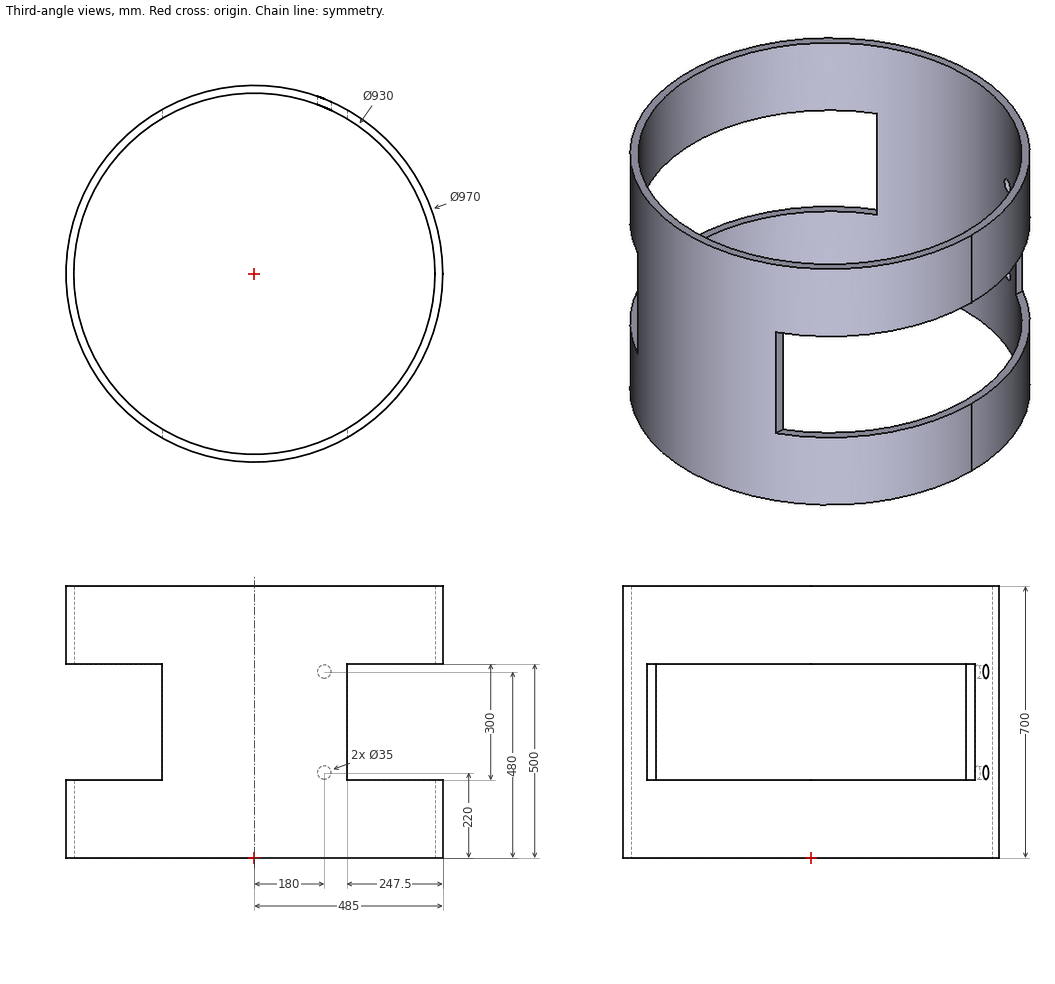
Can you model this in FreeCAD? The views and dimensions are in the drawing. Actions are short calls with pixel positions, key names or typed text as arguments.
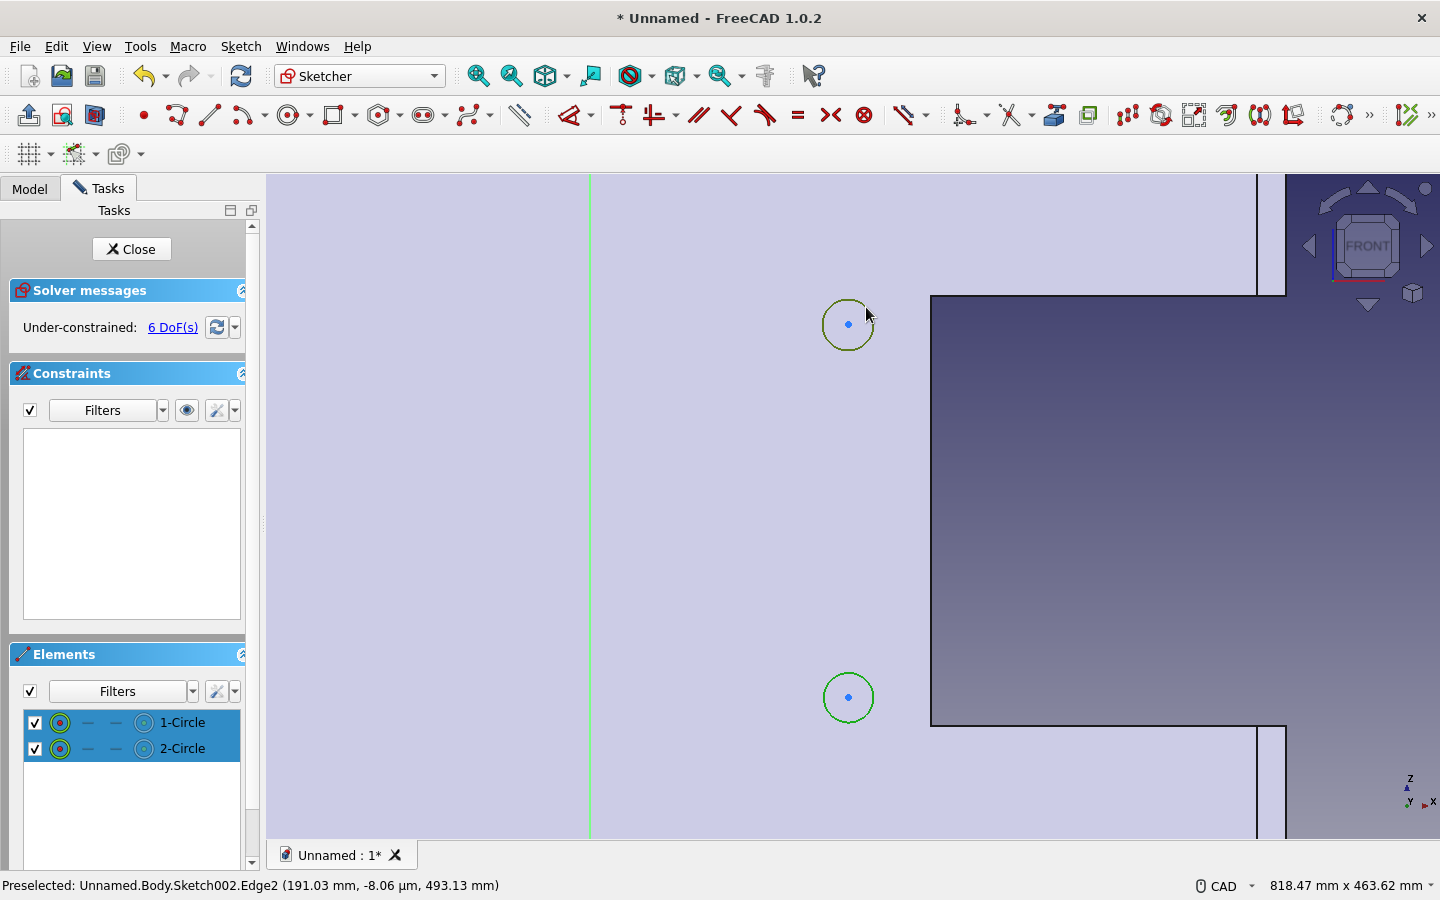
key(e)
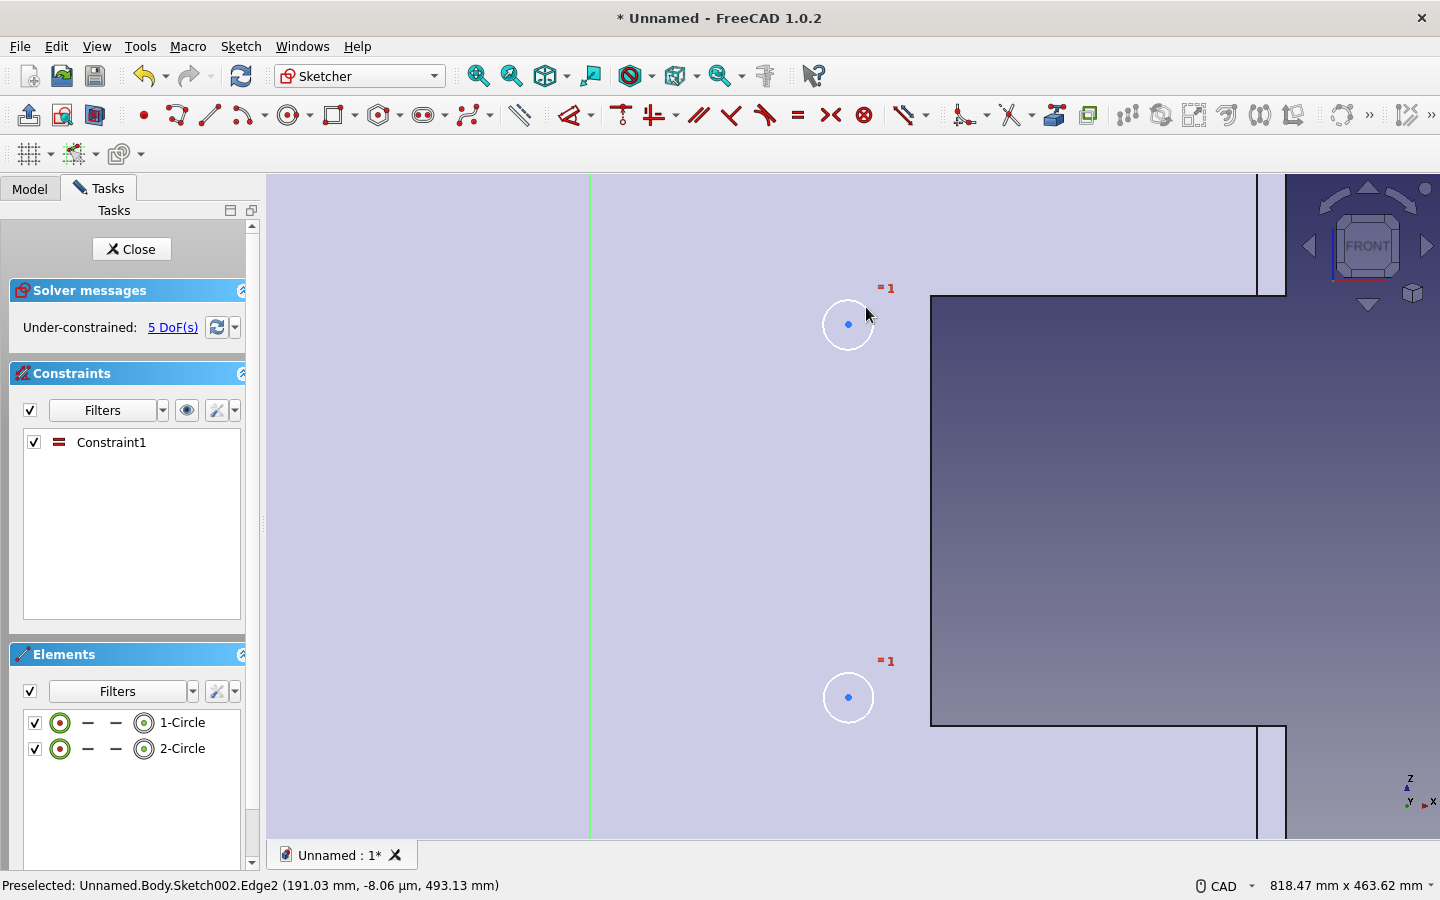
click(849, 698)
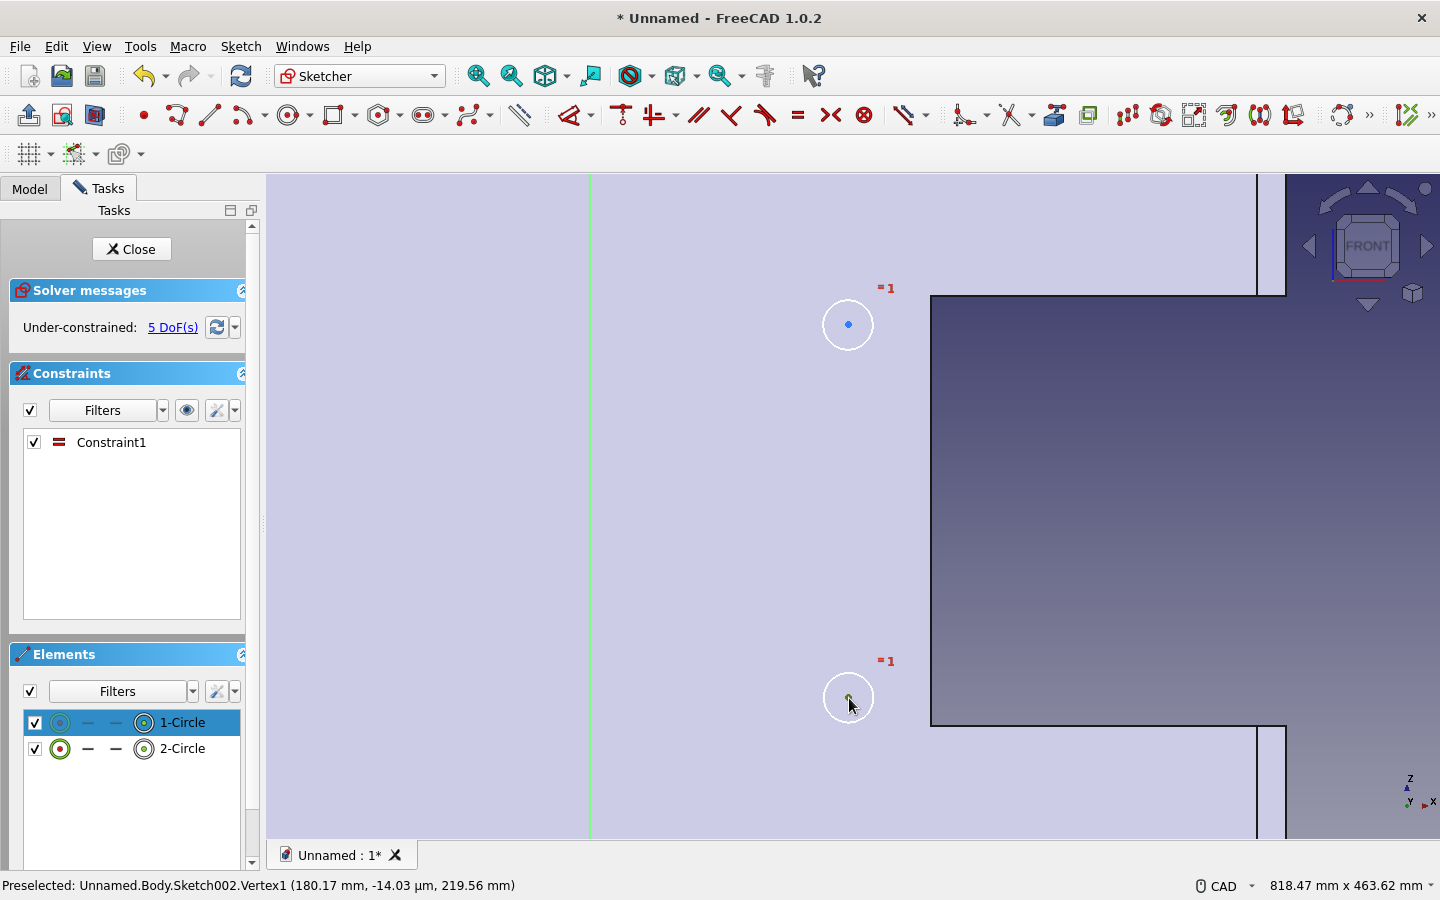
click(848, 325)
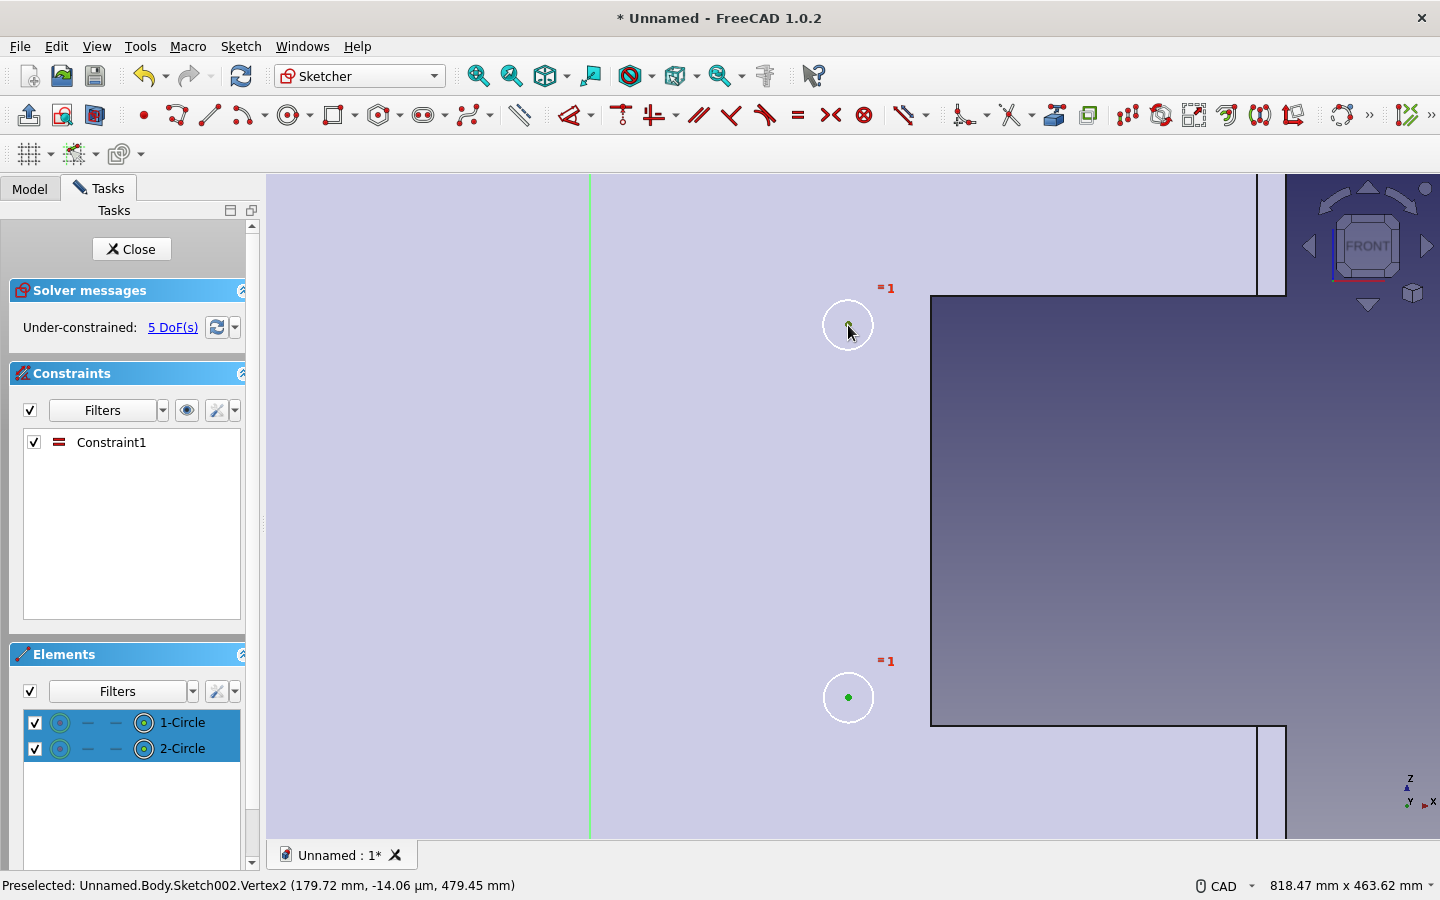
key(v)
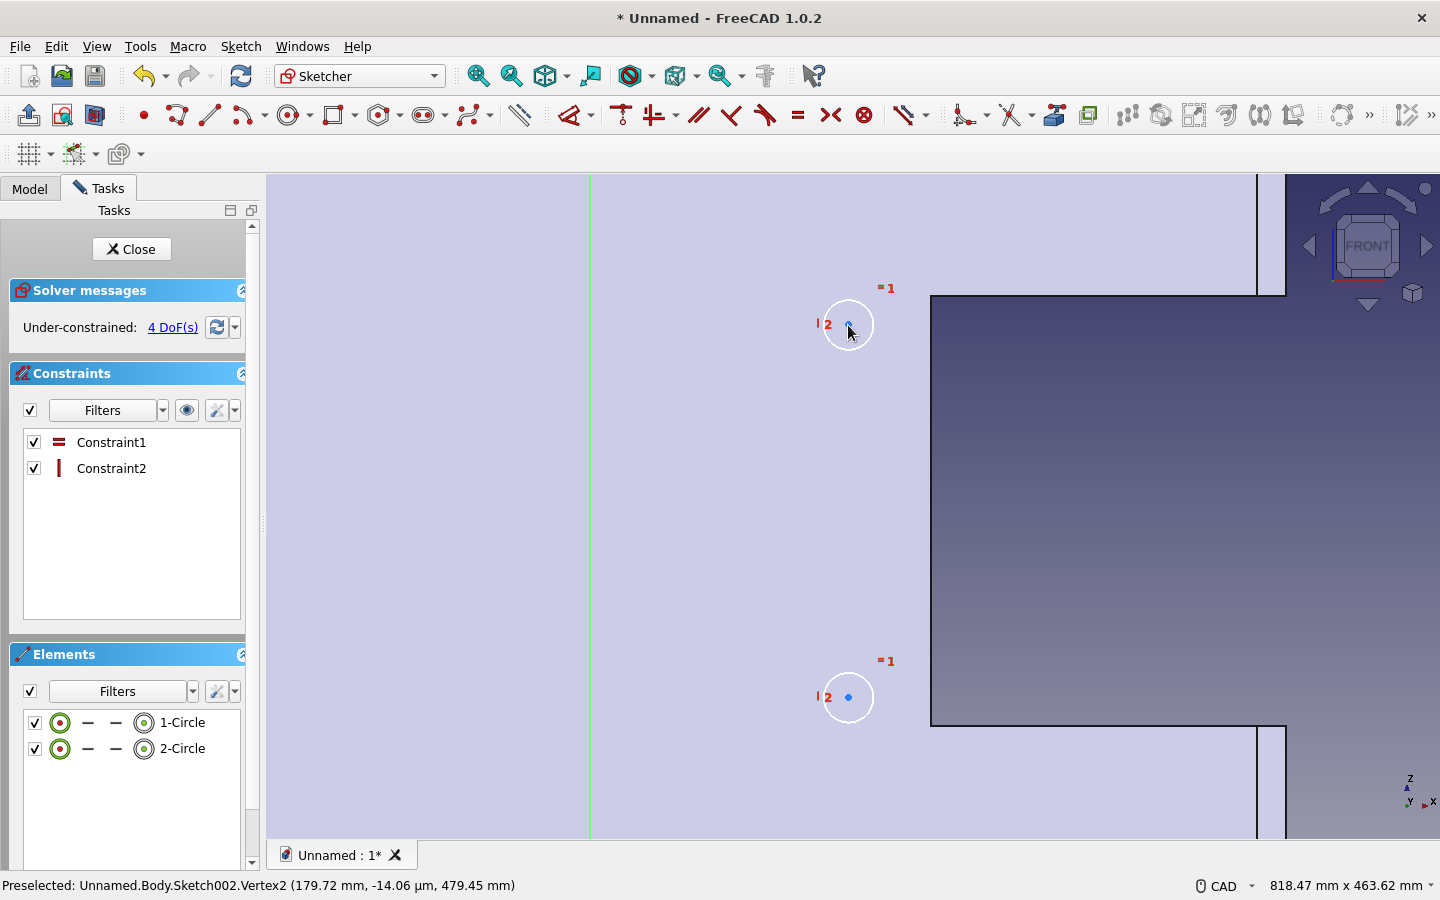
key(d)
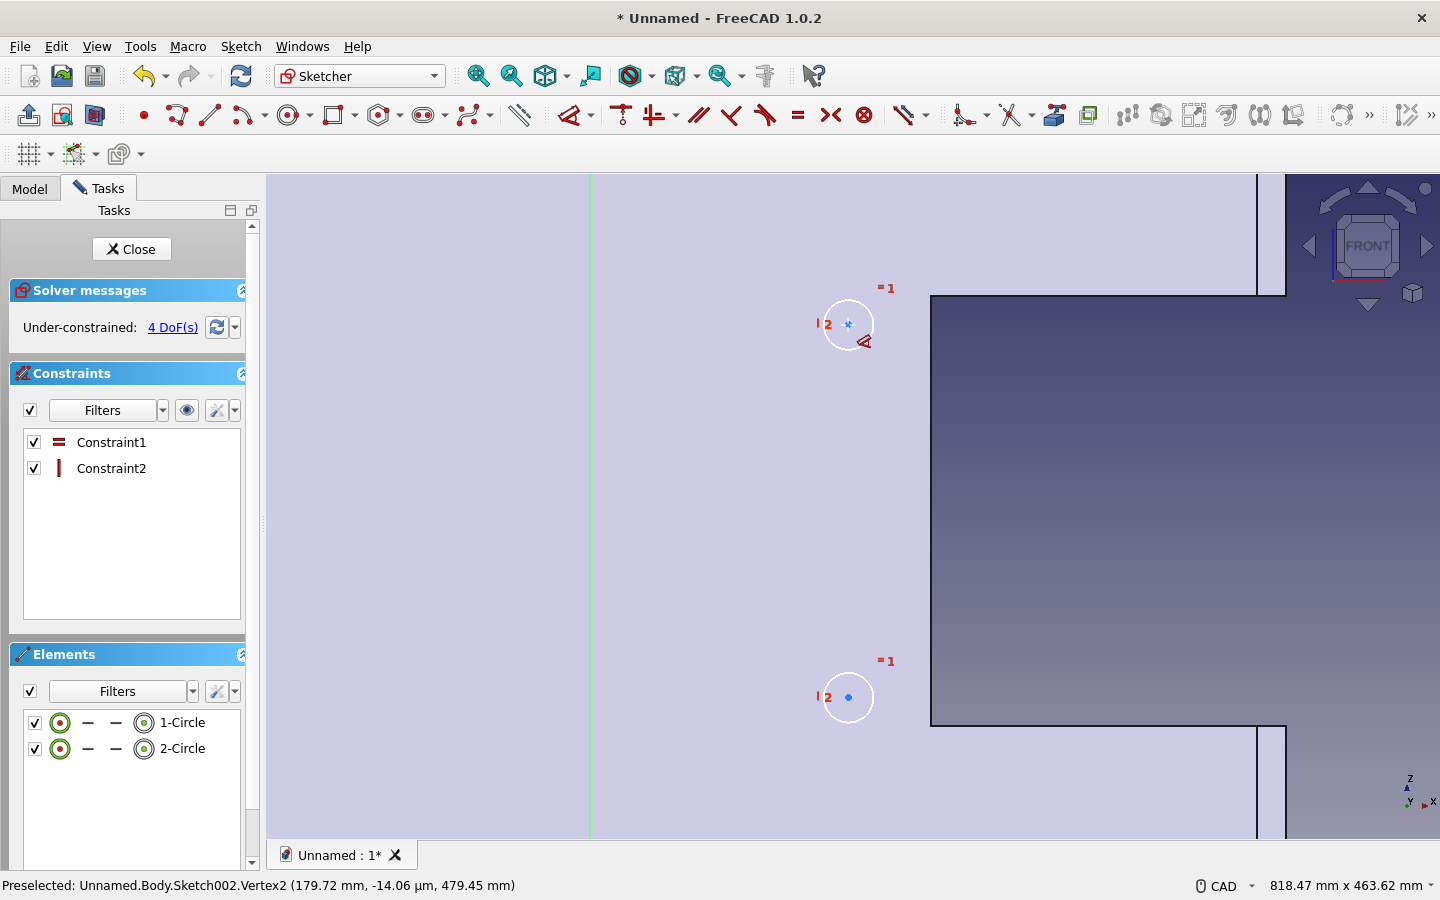
click(866, 680)
click(888, 657)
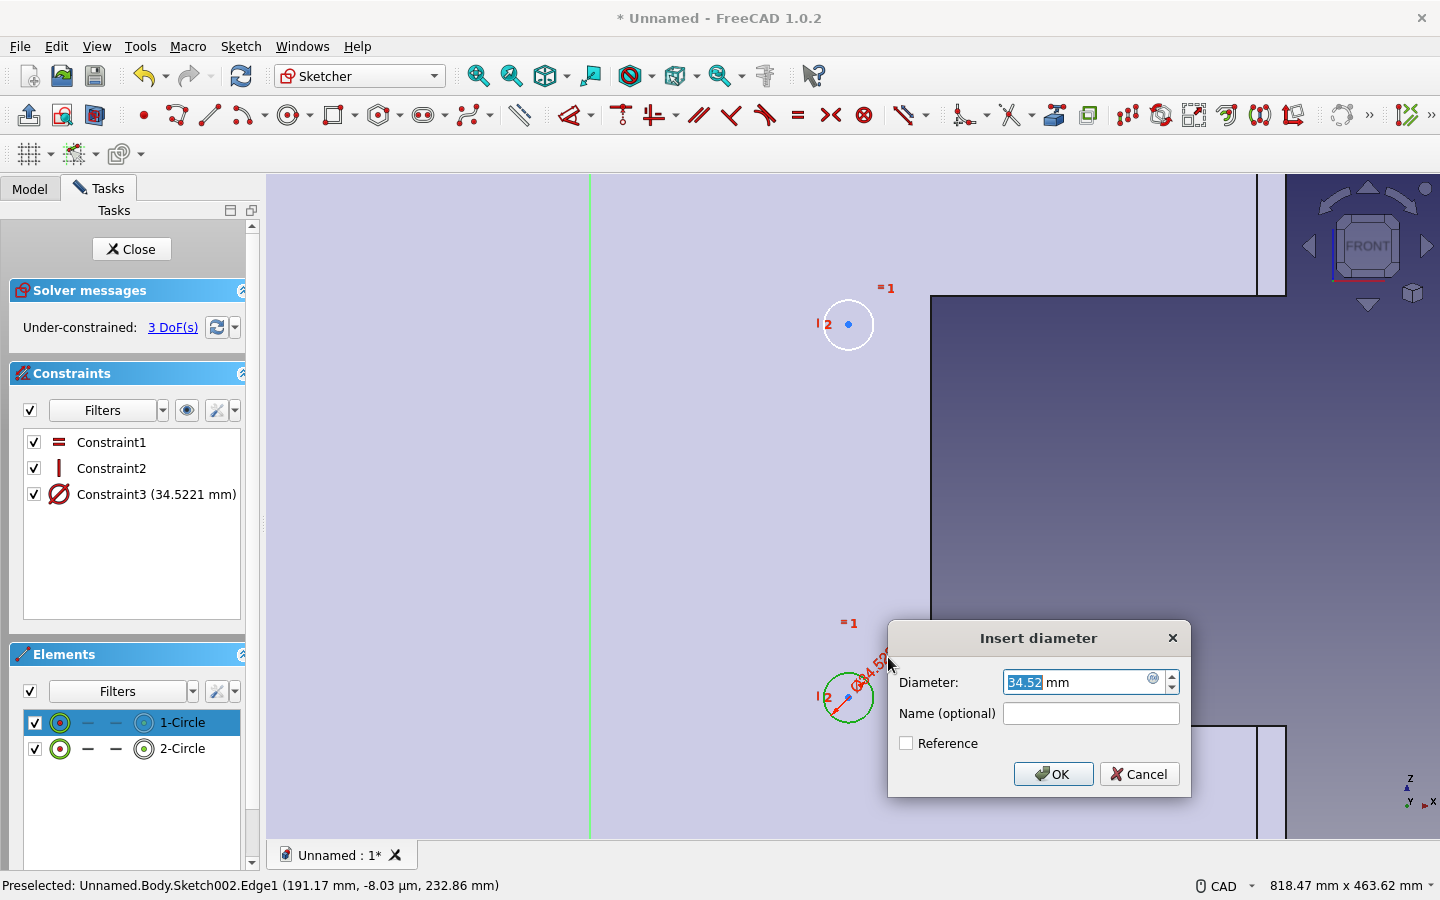
text(35)
key(Return)